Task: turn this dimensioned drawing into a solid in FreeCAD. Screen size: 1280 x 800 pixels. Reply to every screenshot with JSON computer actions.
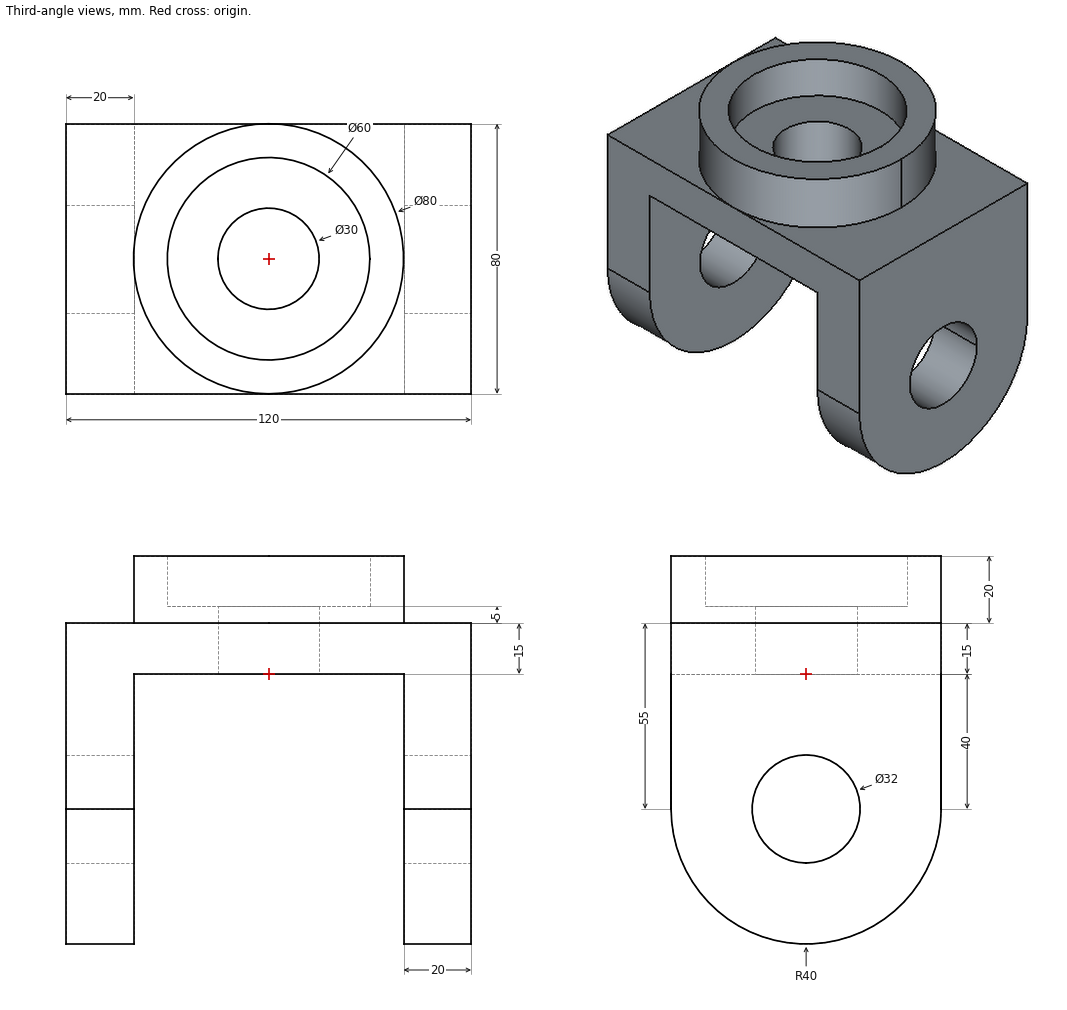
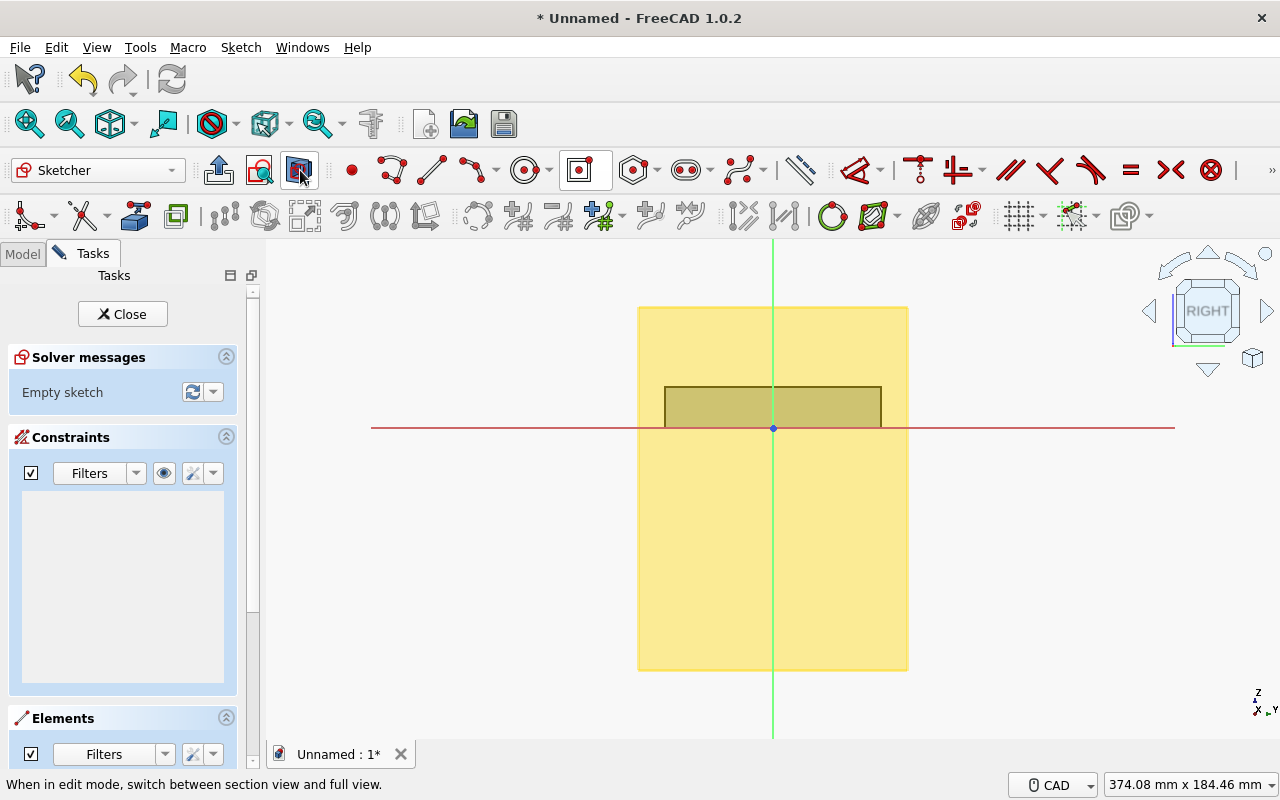
{"action": "left_click", "coordinate": [392, 170]}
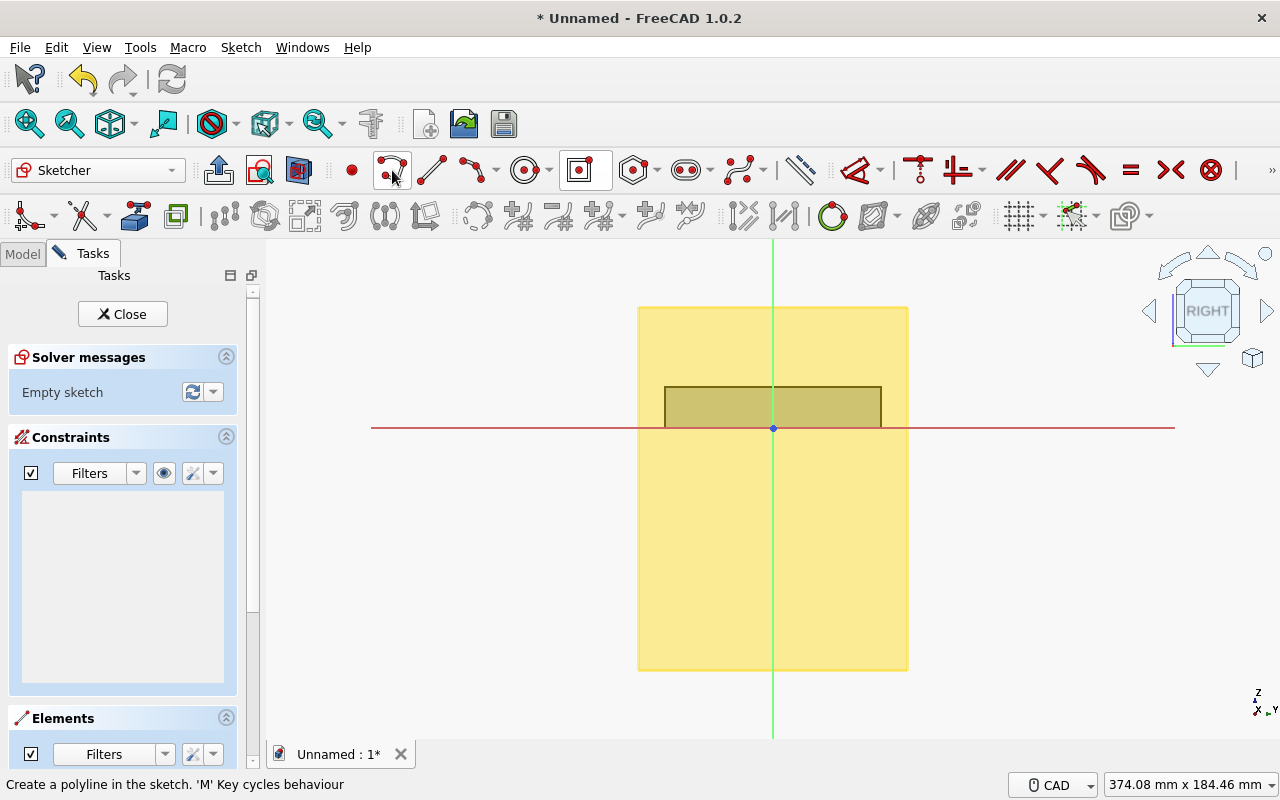
{"action": "left_click", "coordinate": [665, 536]}
{"action": "left_click", "coordinate": [665, 387]}
{"action": "left_click", "coordinate": [881, 387]}
{"action": "left_click", "coordinate": [881, 536]}
{"action": "right_click", "coordinate": [881, 536]}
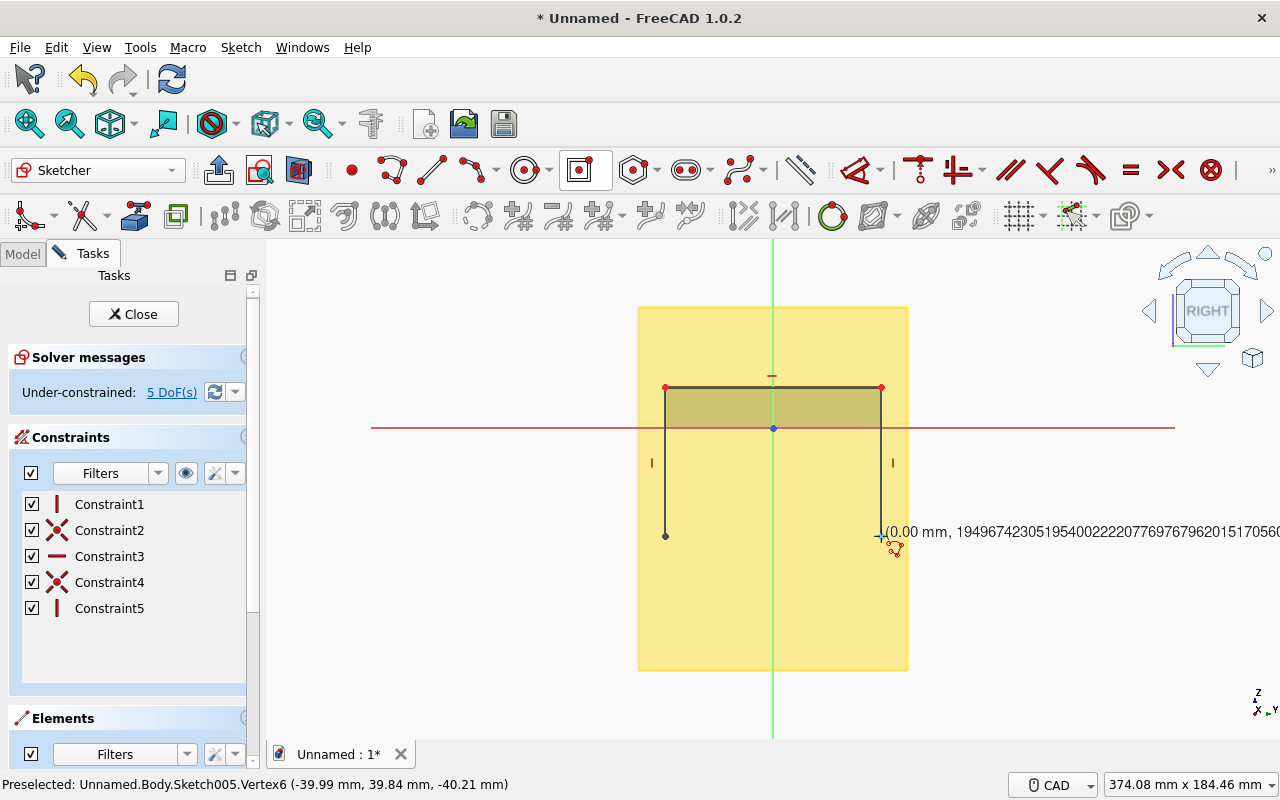
{"action": "left_click", "coordinate": [472, 170]}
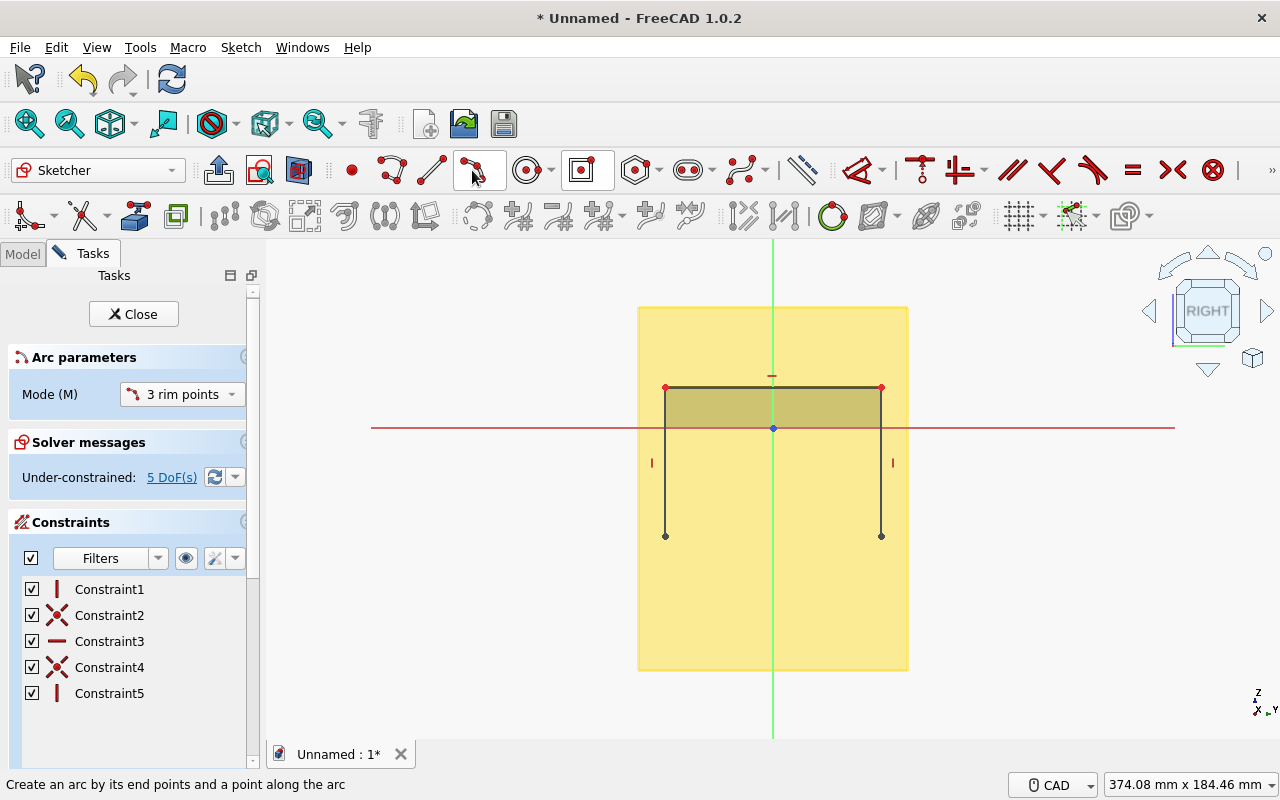
{"action": "left_click", "coordinate": [881, 537]}
{"action": "left_click", "coordinate": [665, 537]}
{"action": "left_click", "coordinate": [739, 640]}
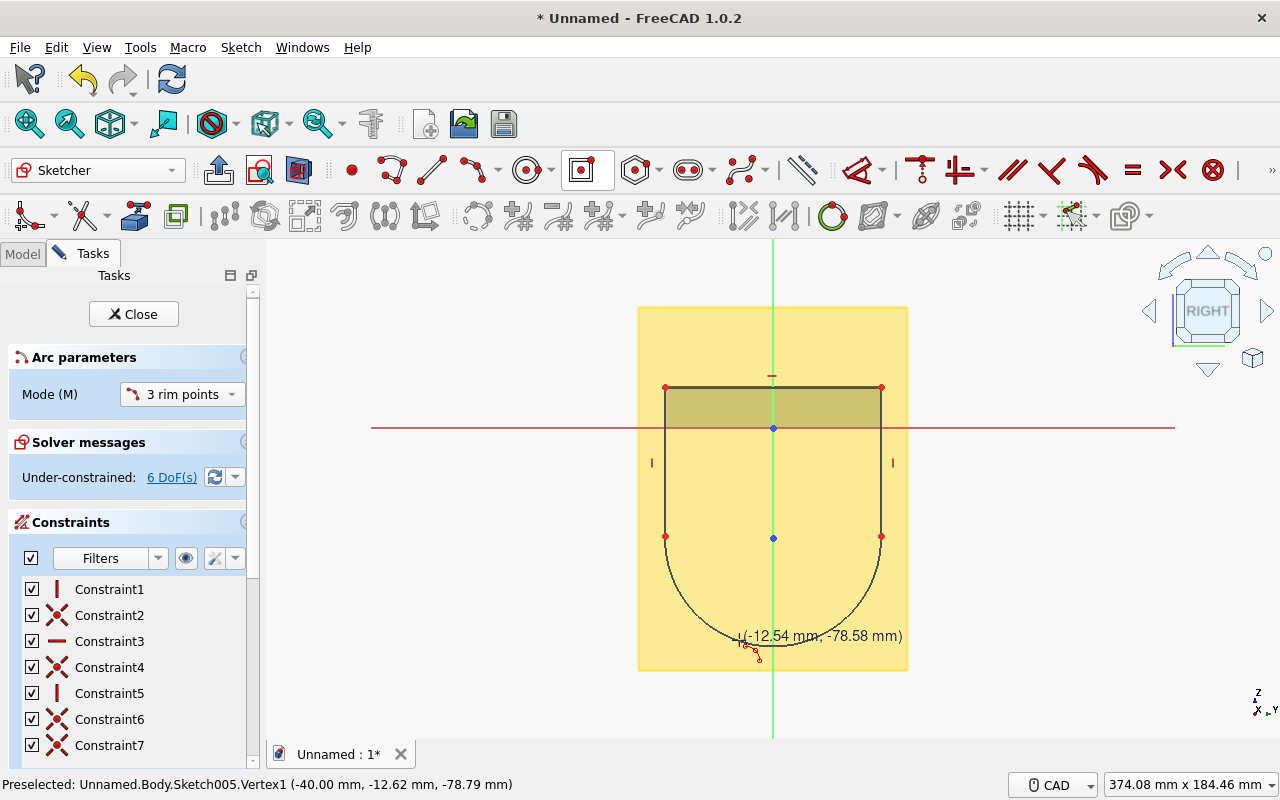
{"action": "key", "text": "g c"}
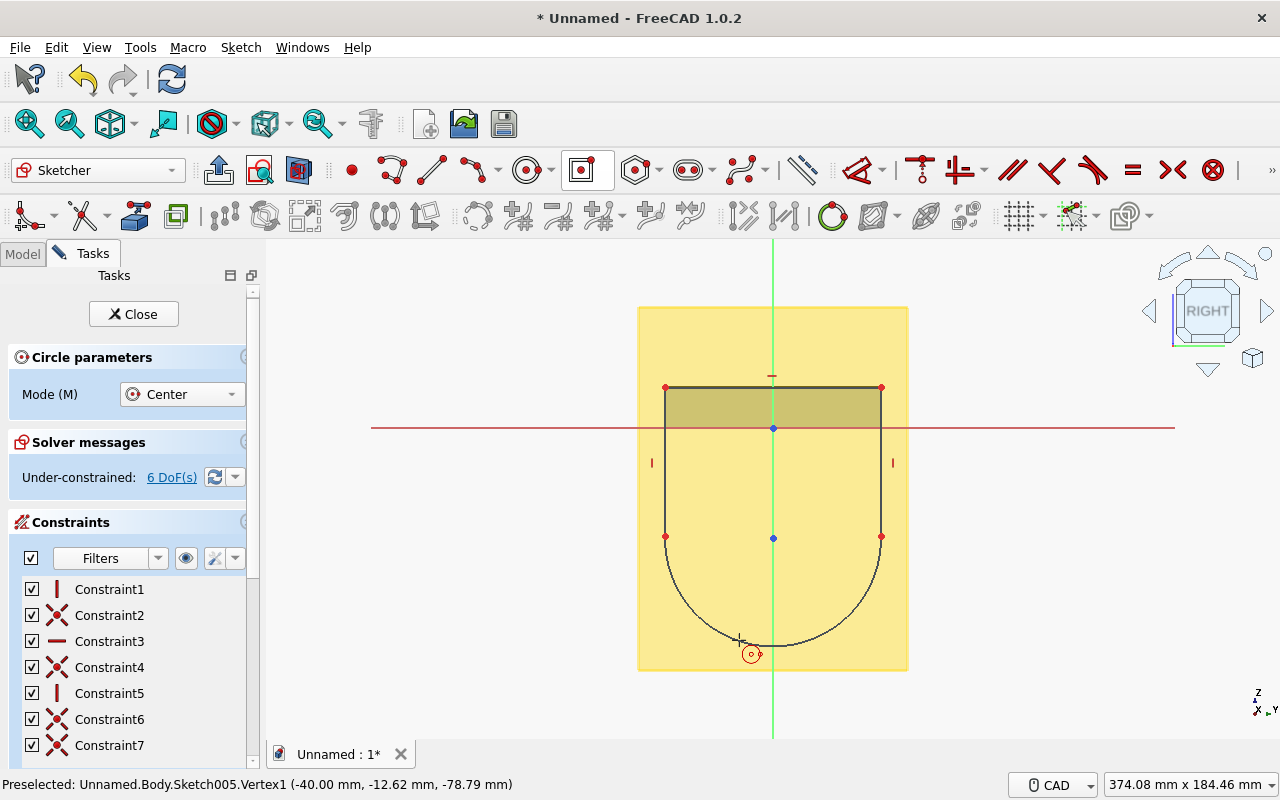
{"action": "left_click", "coordinate": [773, 536]}
{"action": "left_click", "coordinate": [804, 506]}
{"action": "key", "text": "Escape"}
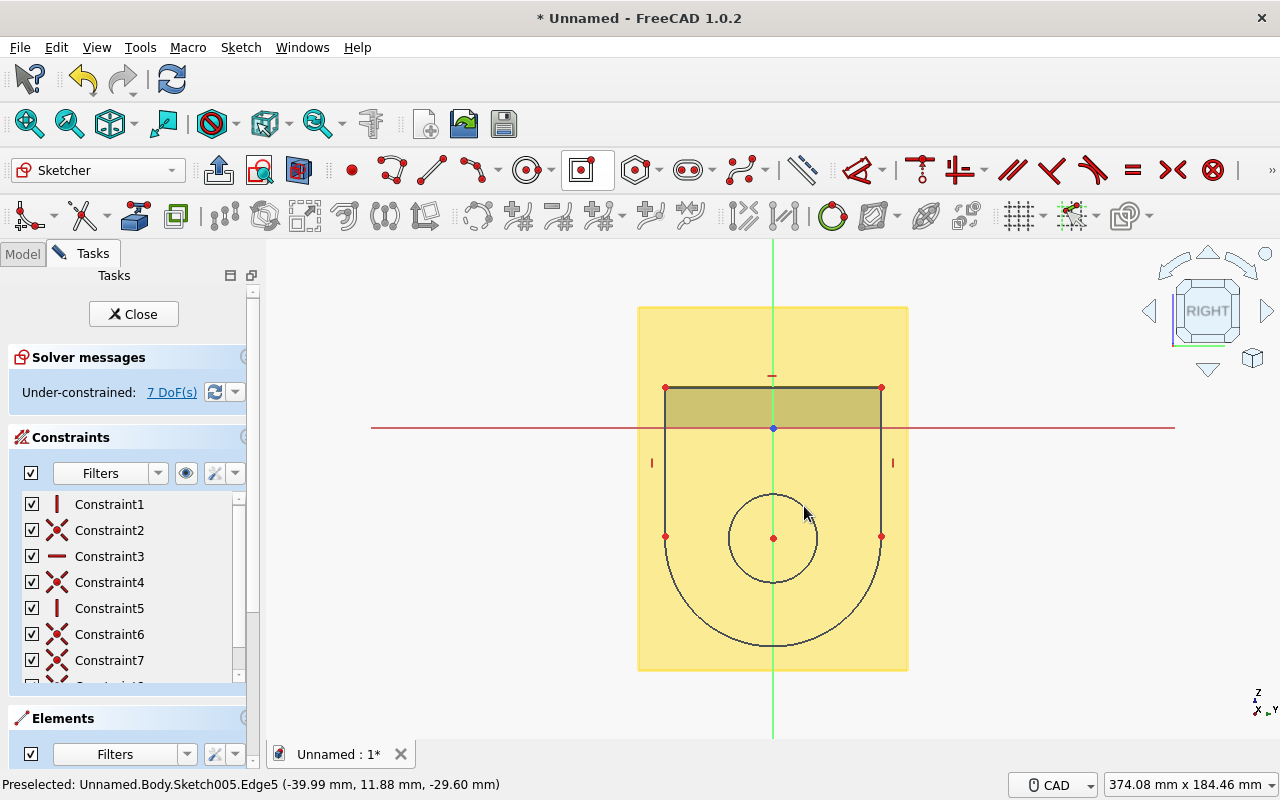
{"action": "left_click", "coordinate": [773, 538]}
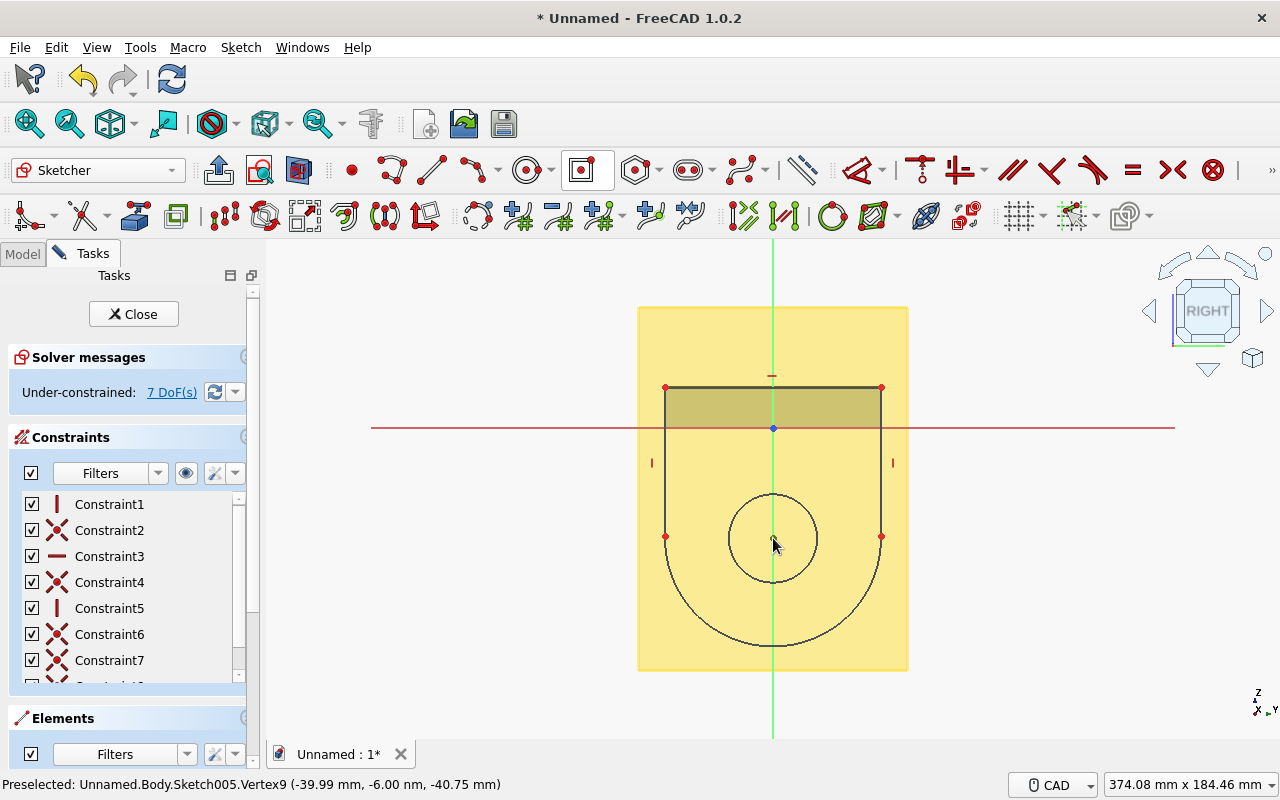
{"action": "left_click", "coordinate": [773, 679]}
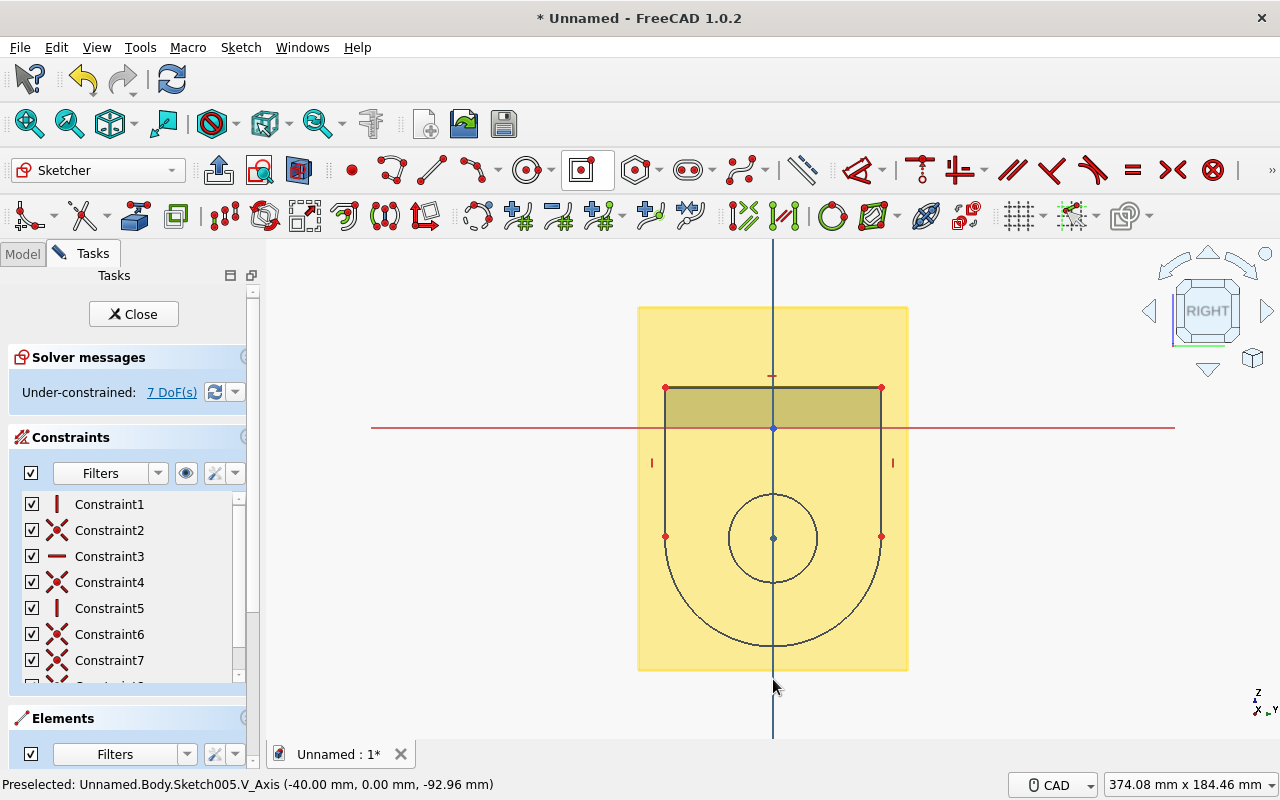
{"action": "left_click", "coordinate": [920, 170]}